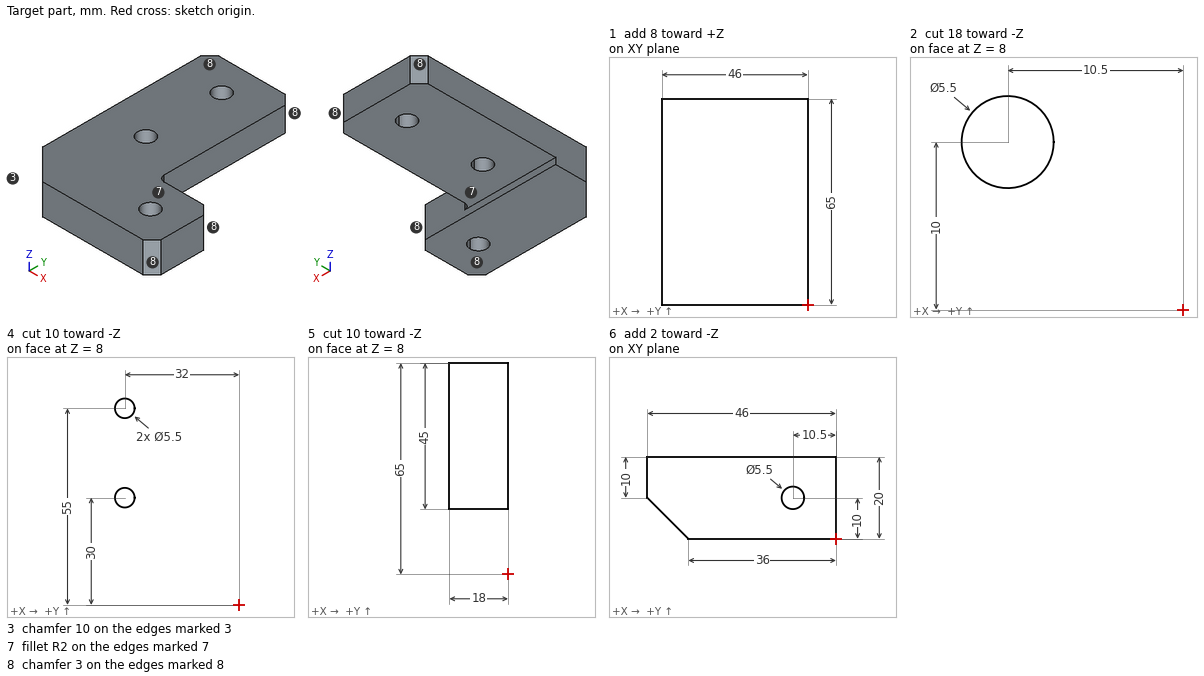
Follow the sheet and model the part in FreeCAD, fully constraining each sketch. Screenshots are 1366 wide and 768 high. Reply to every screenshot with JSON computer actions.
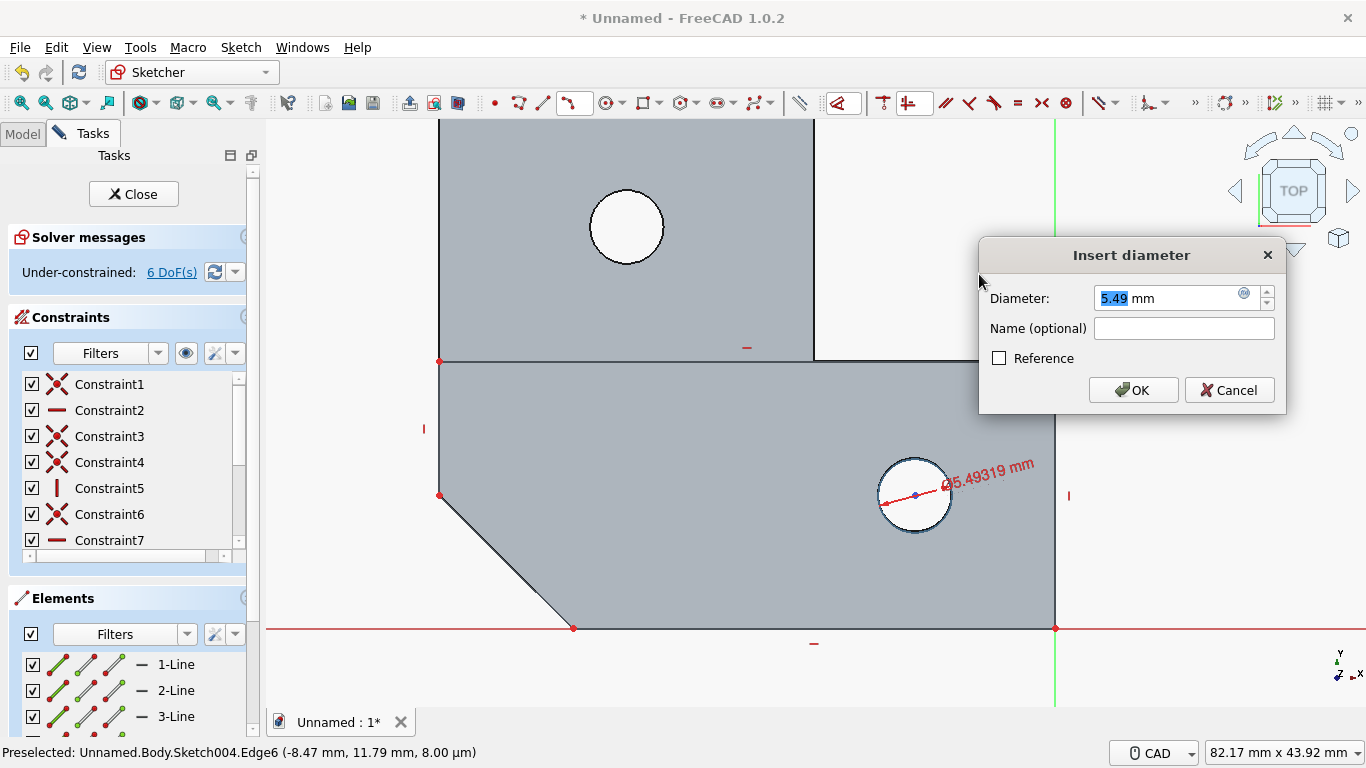
{"action": "type", "text": "5.5"}
{"action": "key", "text": "Return"}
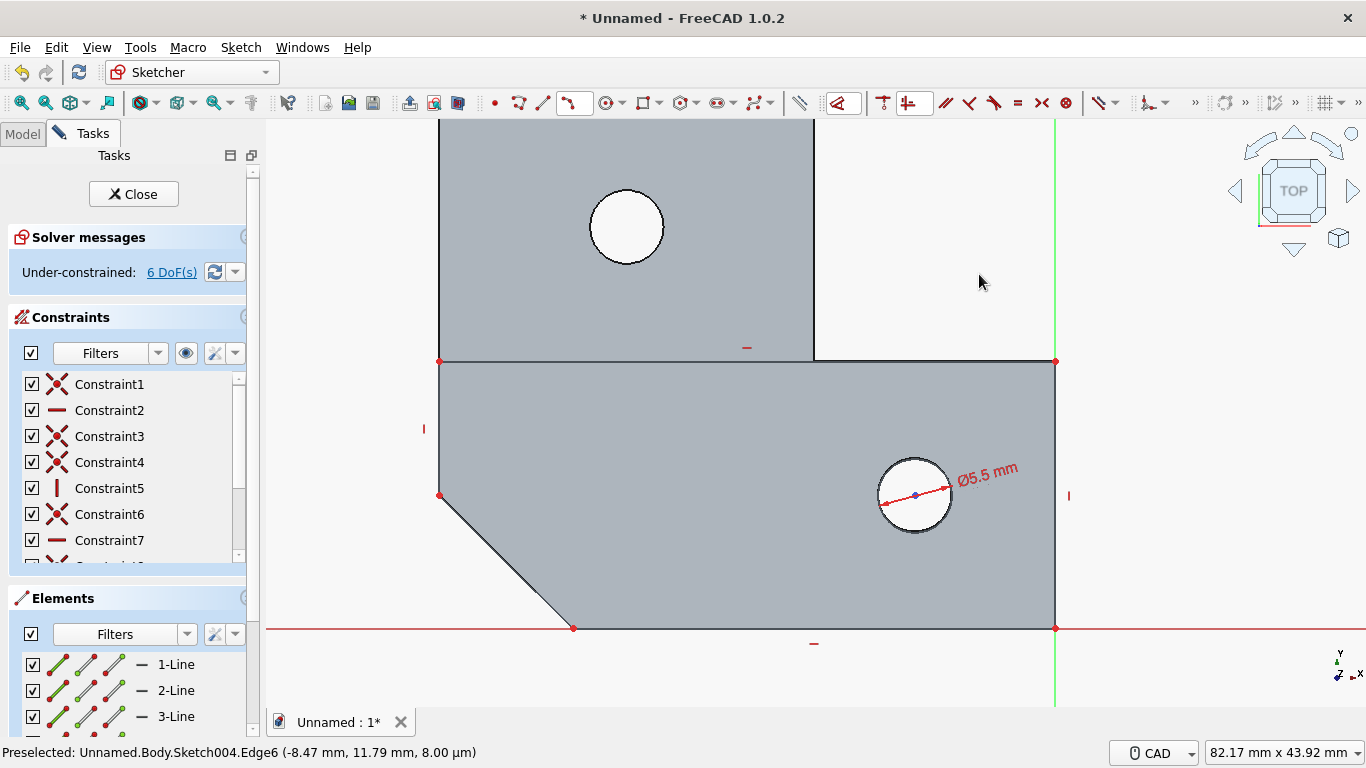
{"action": "left_click", "coordinate": [911, 629]}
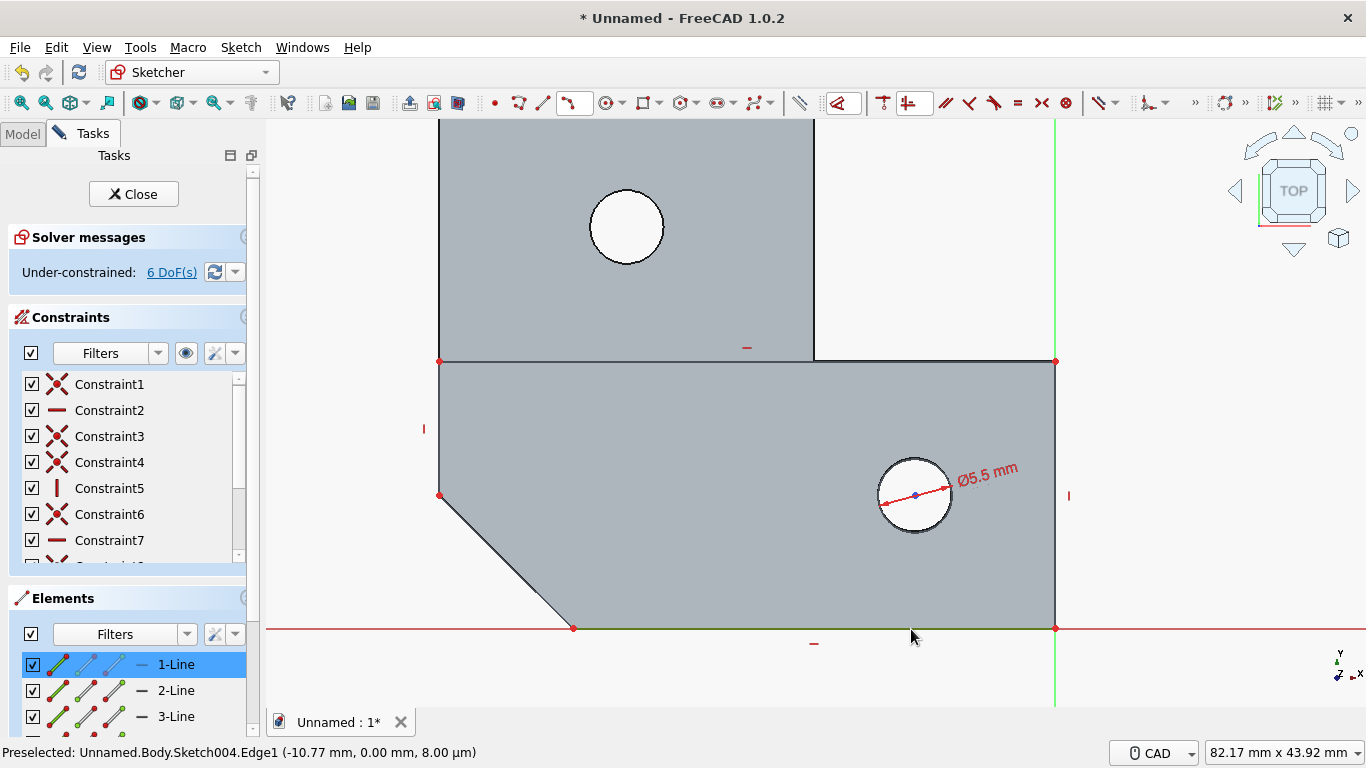
{"action": "key", "text": "l"}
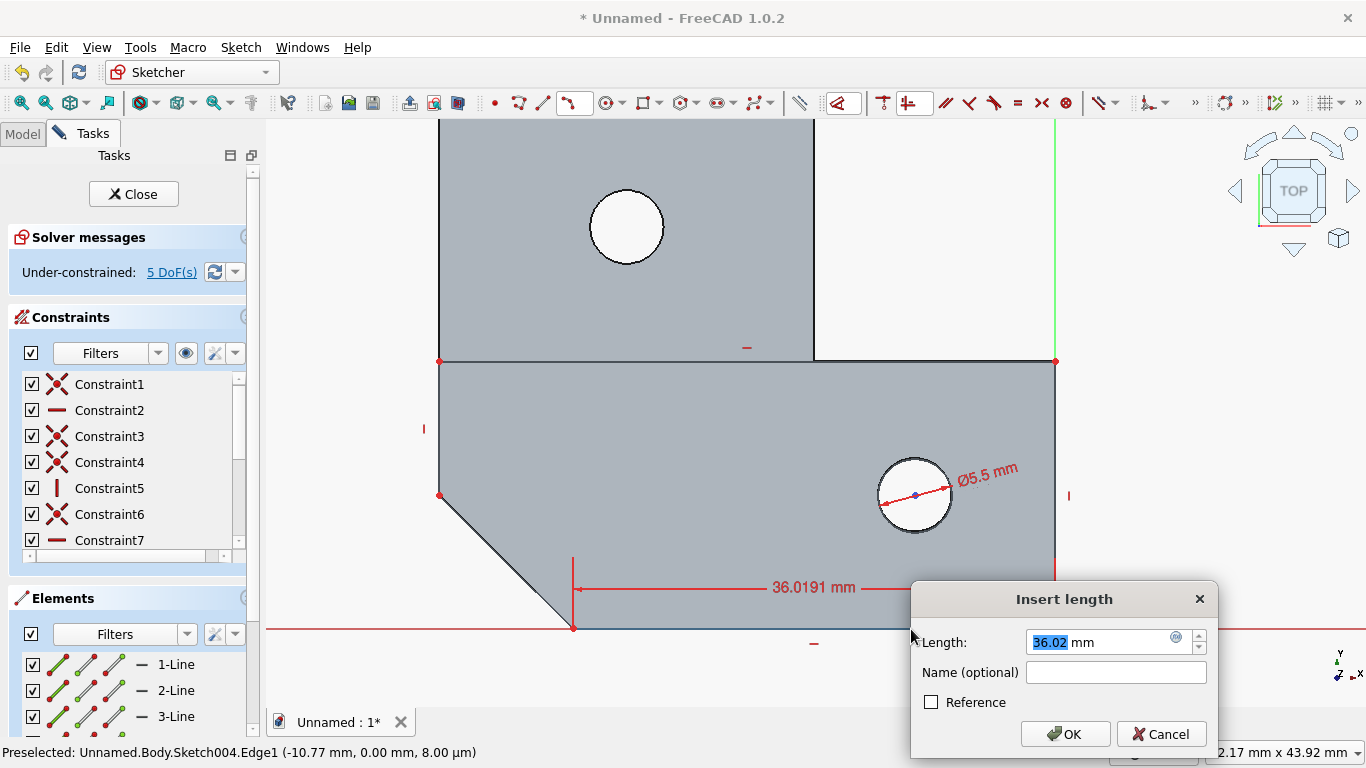
{"action": "type", "text": "36"}
{"action": "key", "text": "Return"}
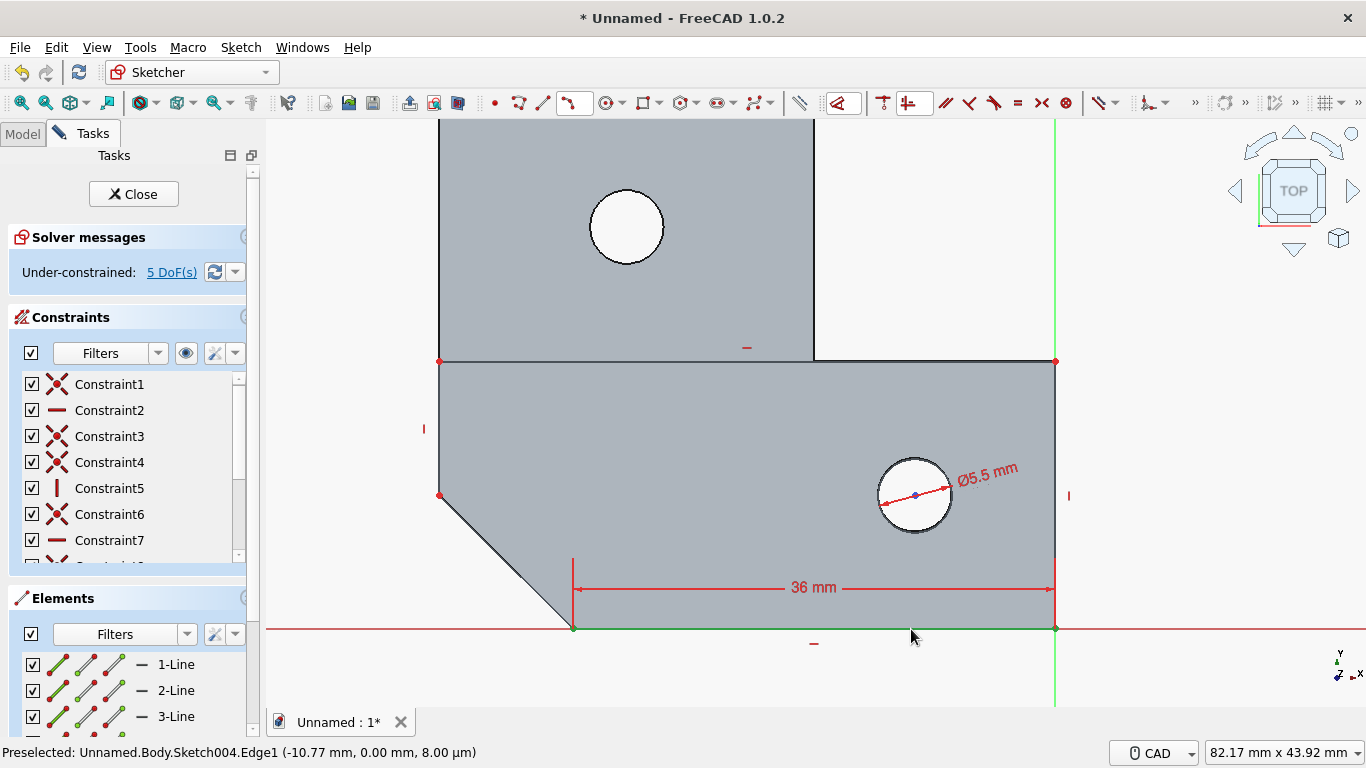
{"action": "left_click", "coordinate": [439, 456]}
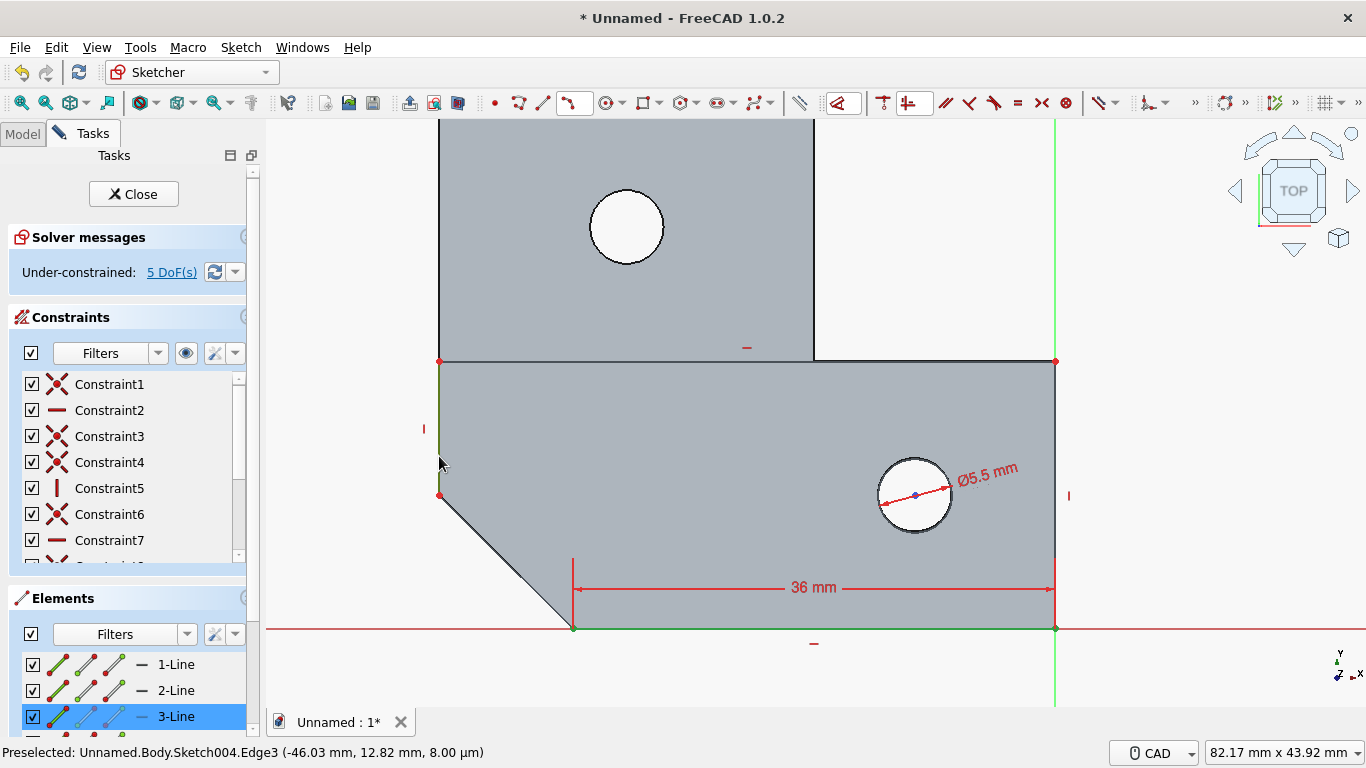
{"action": "key", "text": "i"}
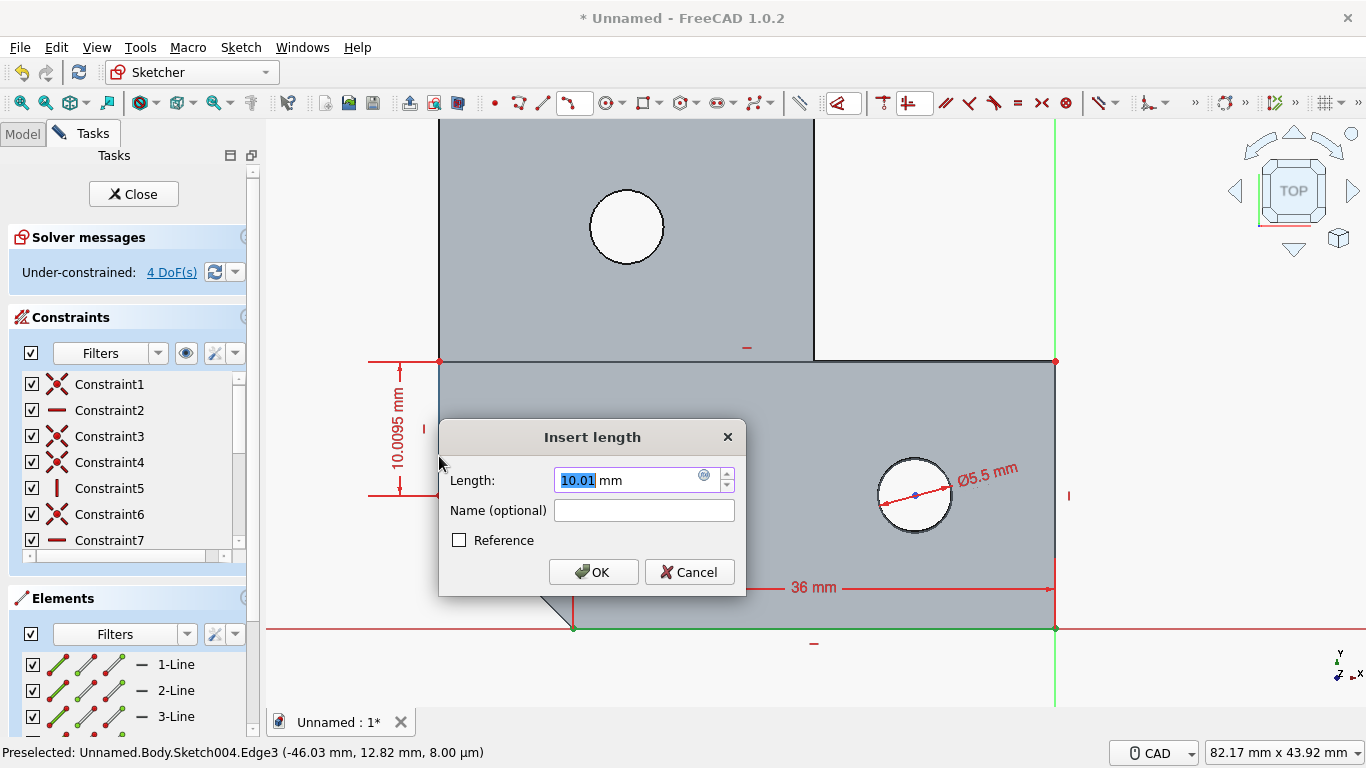
{"action": "type", "text": "10"}
{"action": "key", "text": "Return"}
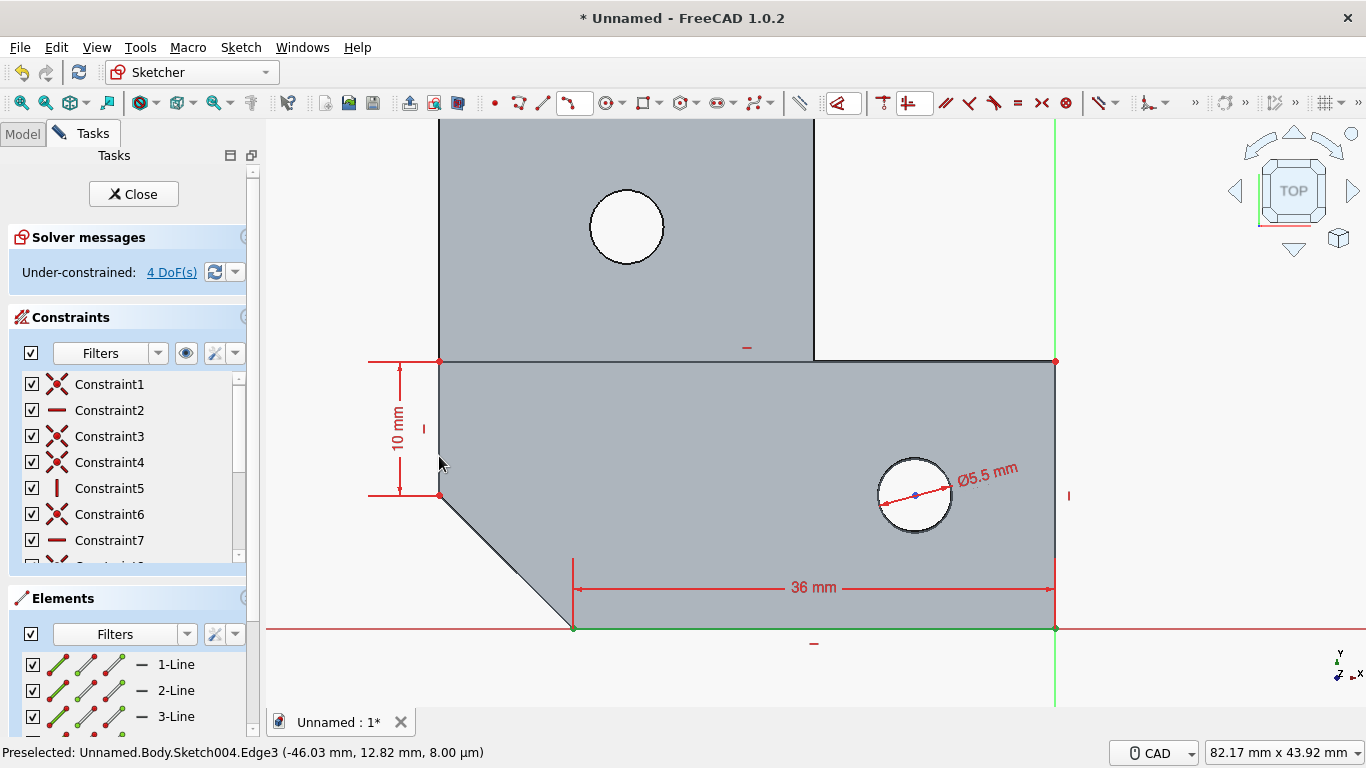
{"action": "left_click", "coordinate": [624, 362]}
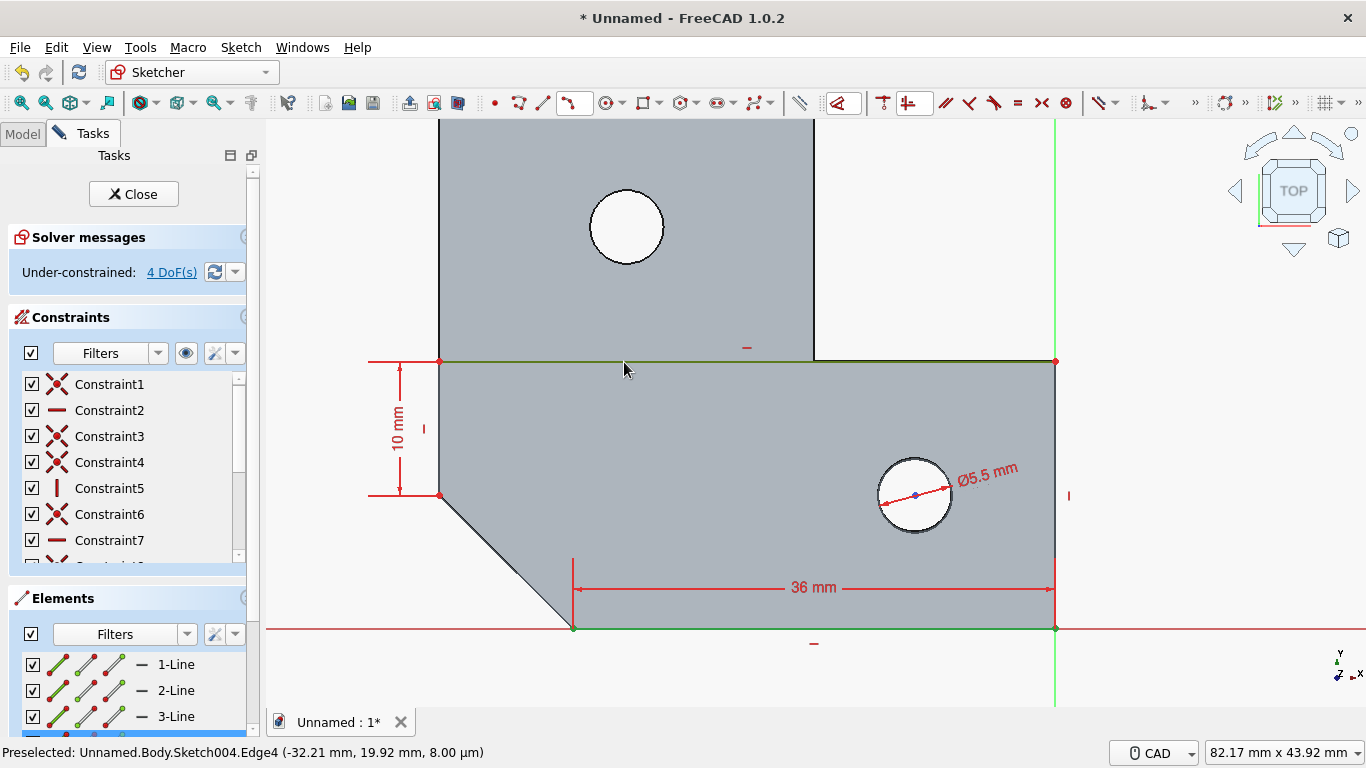
{"action": "key", "text": "l"}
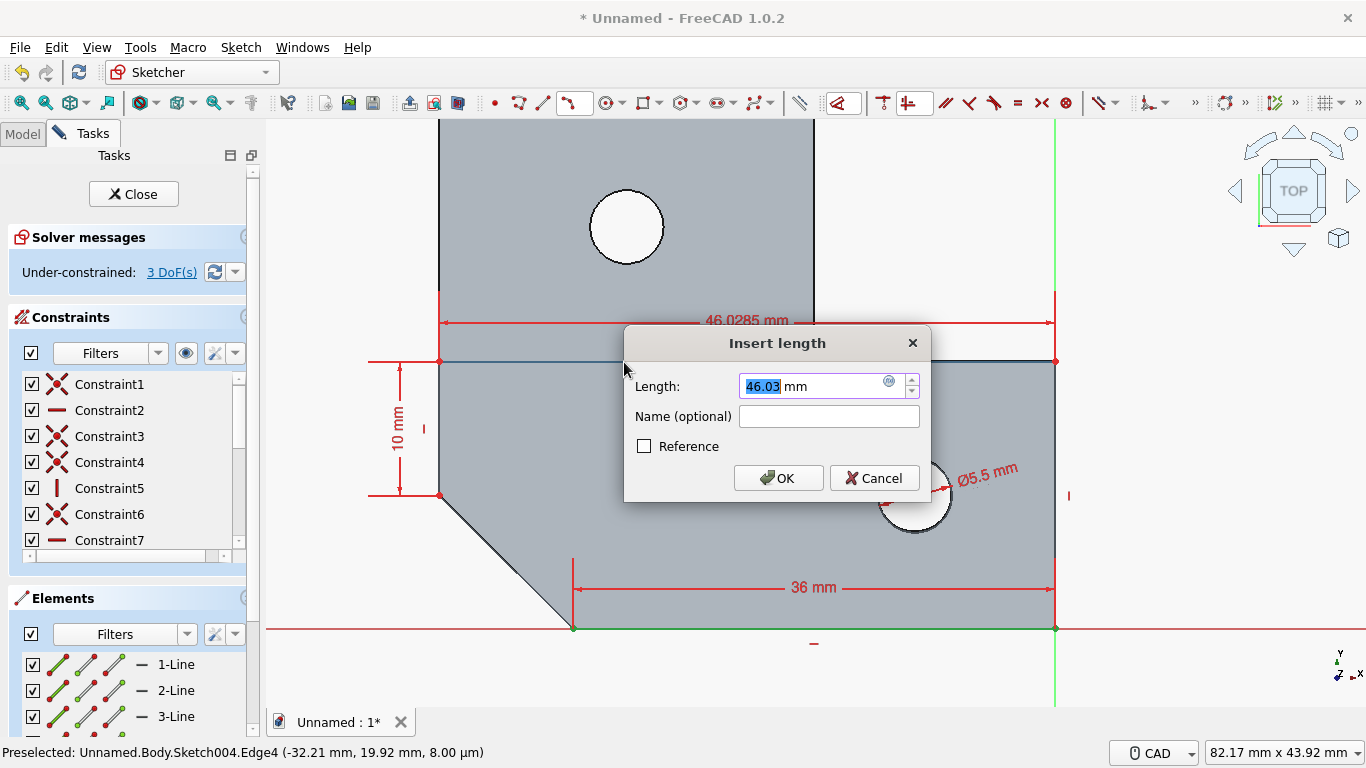
{"action": "type", "text": "46"}
{"action": "key", "text": "Return"}